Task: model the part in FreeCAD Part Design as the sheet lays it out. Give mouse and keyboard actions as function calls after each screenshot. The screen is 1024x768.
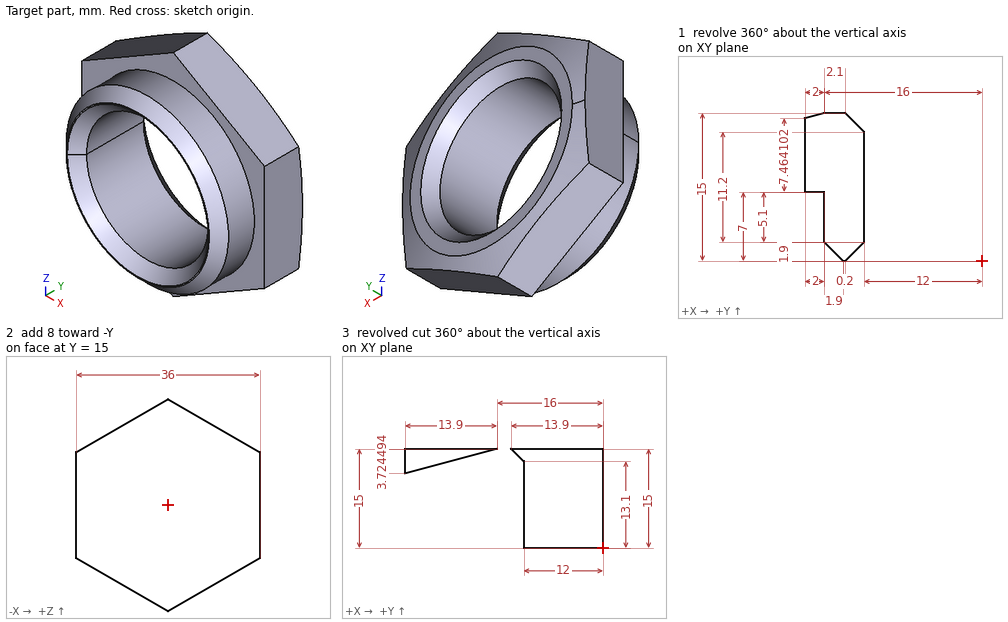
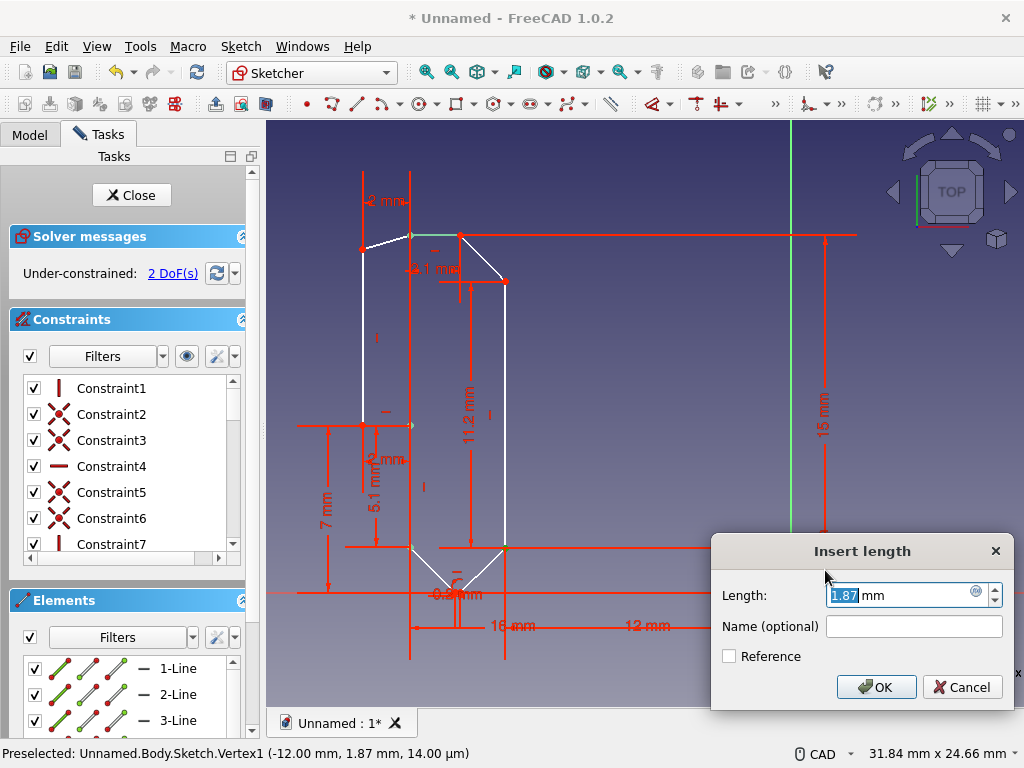
text(1.9)
key(Return)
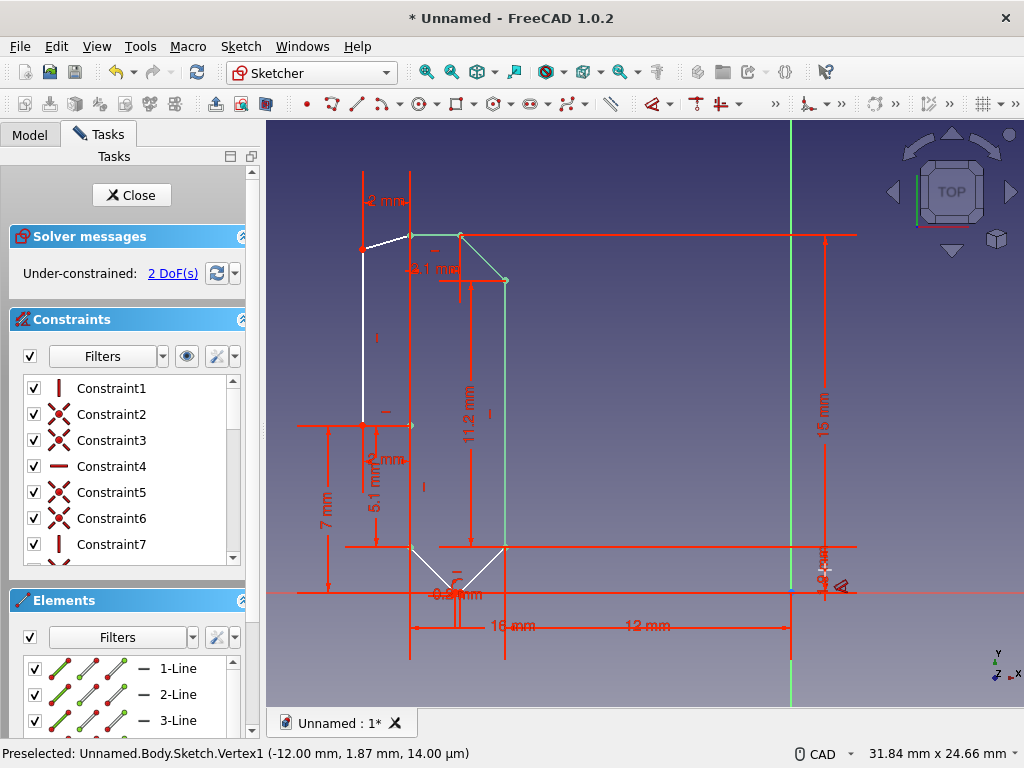
click(424, 561)
click(433, 627)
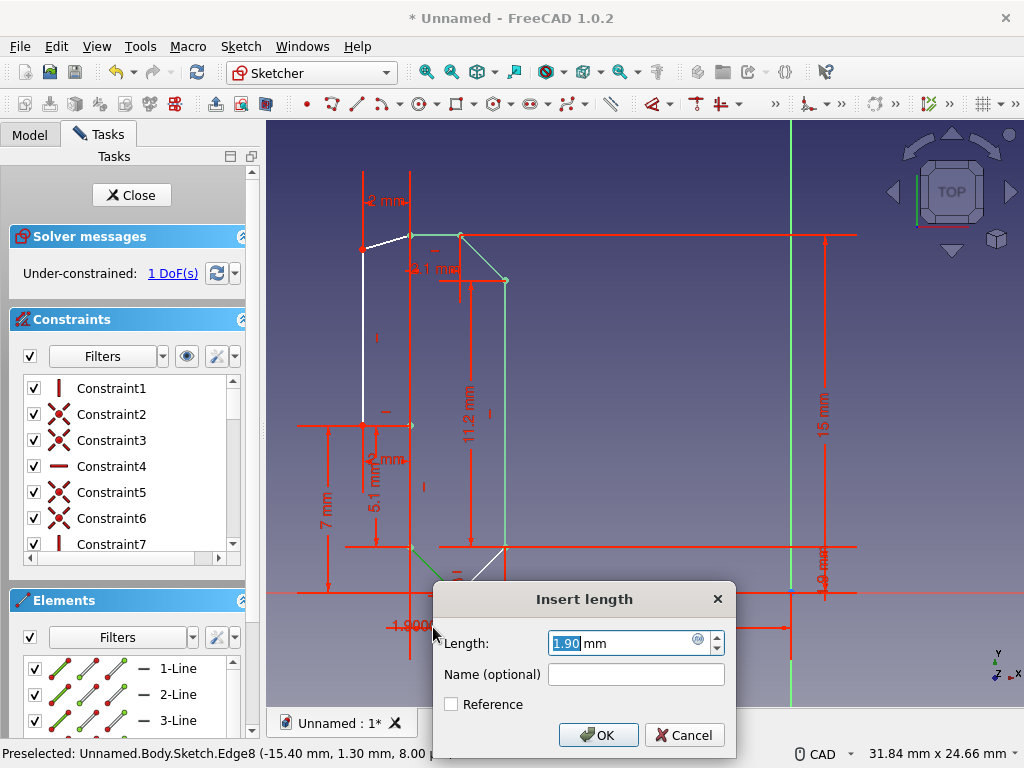
text(1.9)
key(Return)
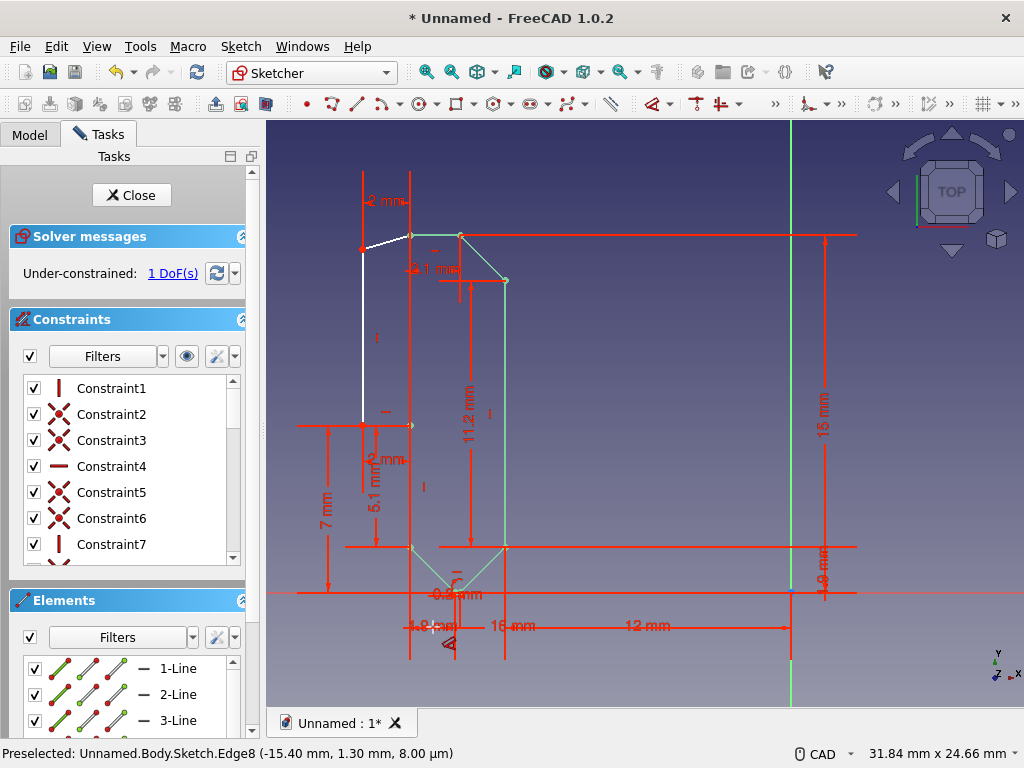
click(363, 302)
click(329, 338)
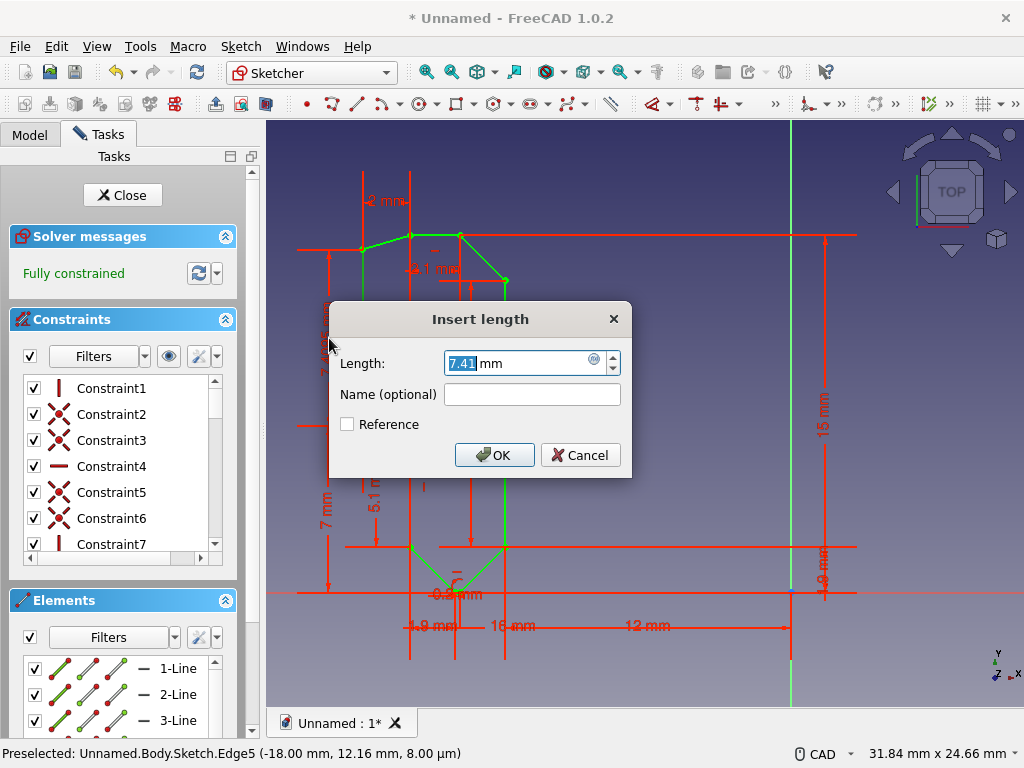
text(7.464102)
key(Return)
key(Escape)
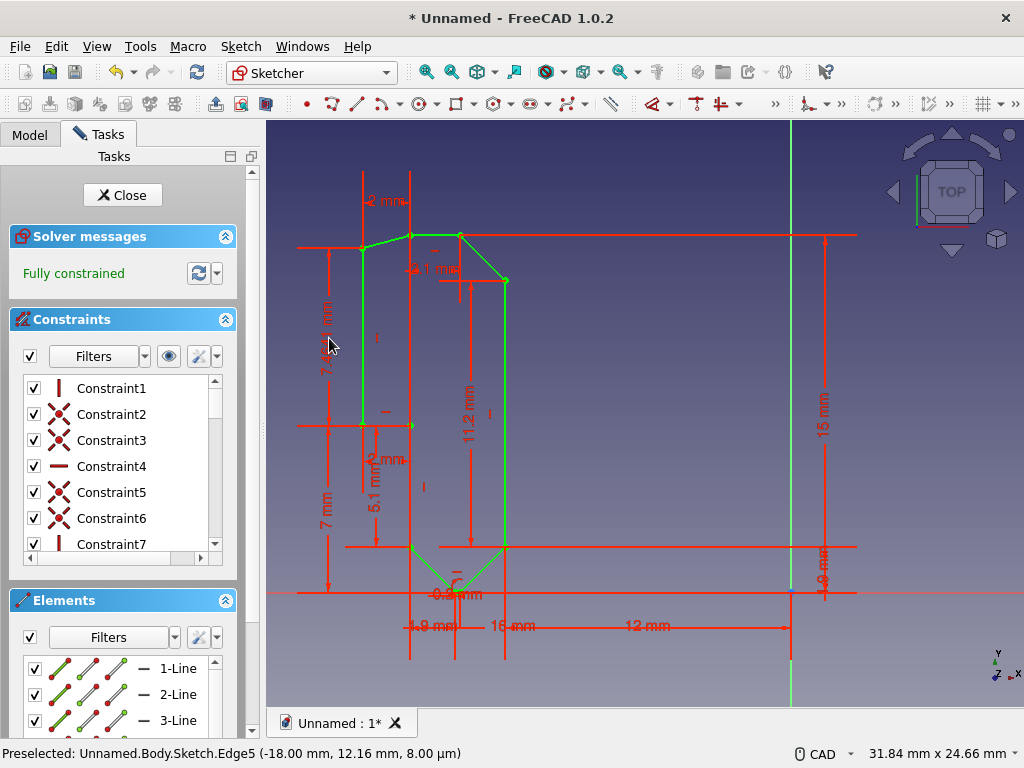
click(123, 195)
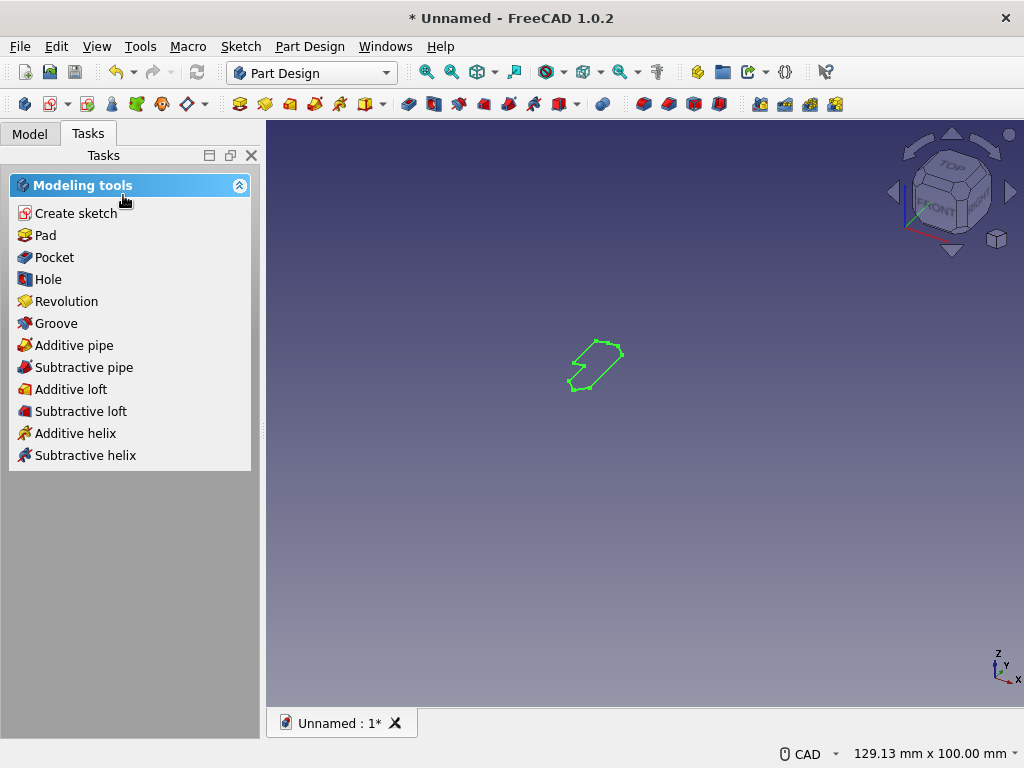
click(265, 104)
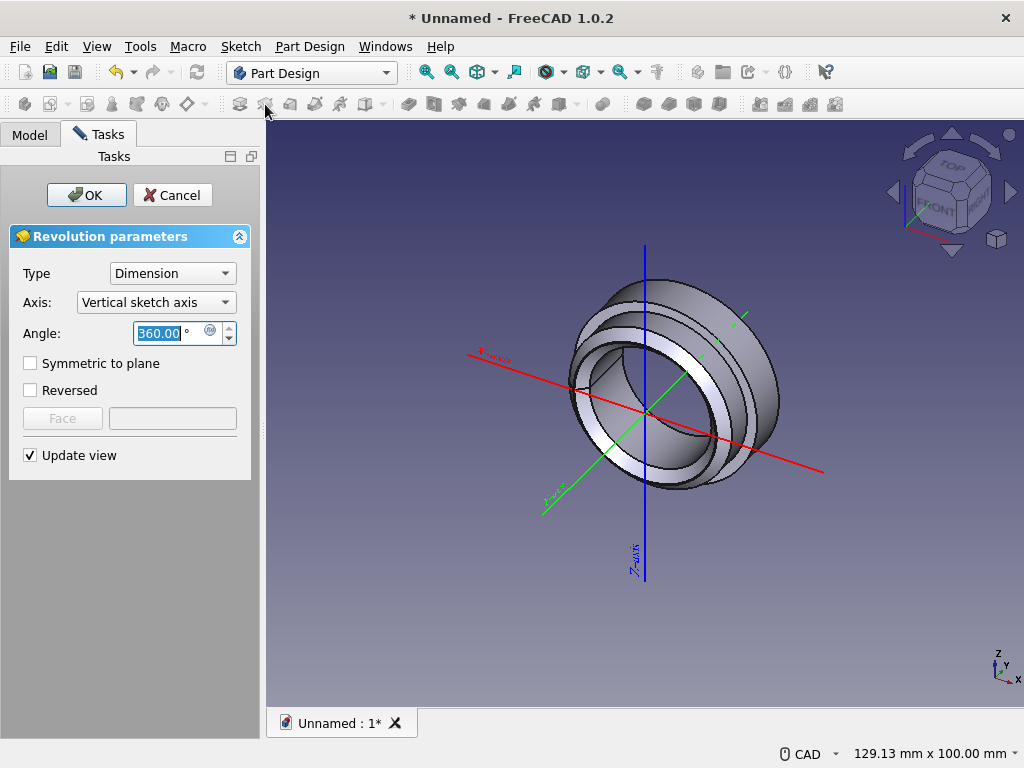
click(87, 195)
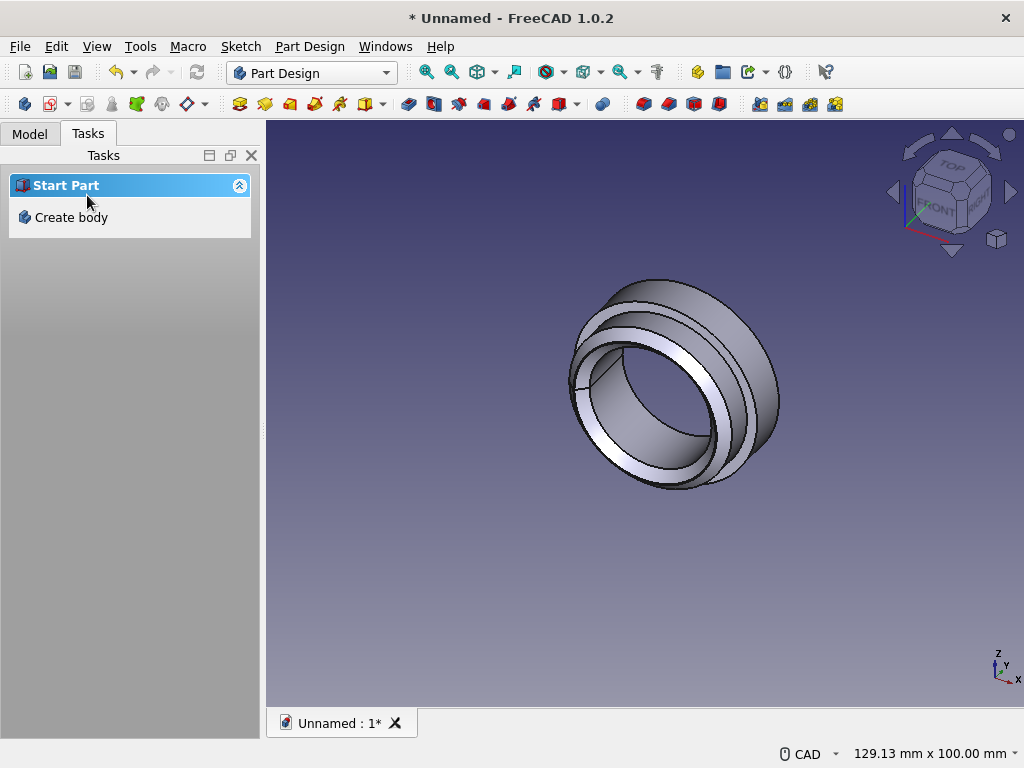
key(4)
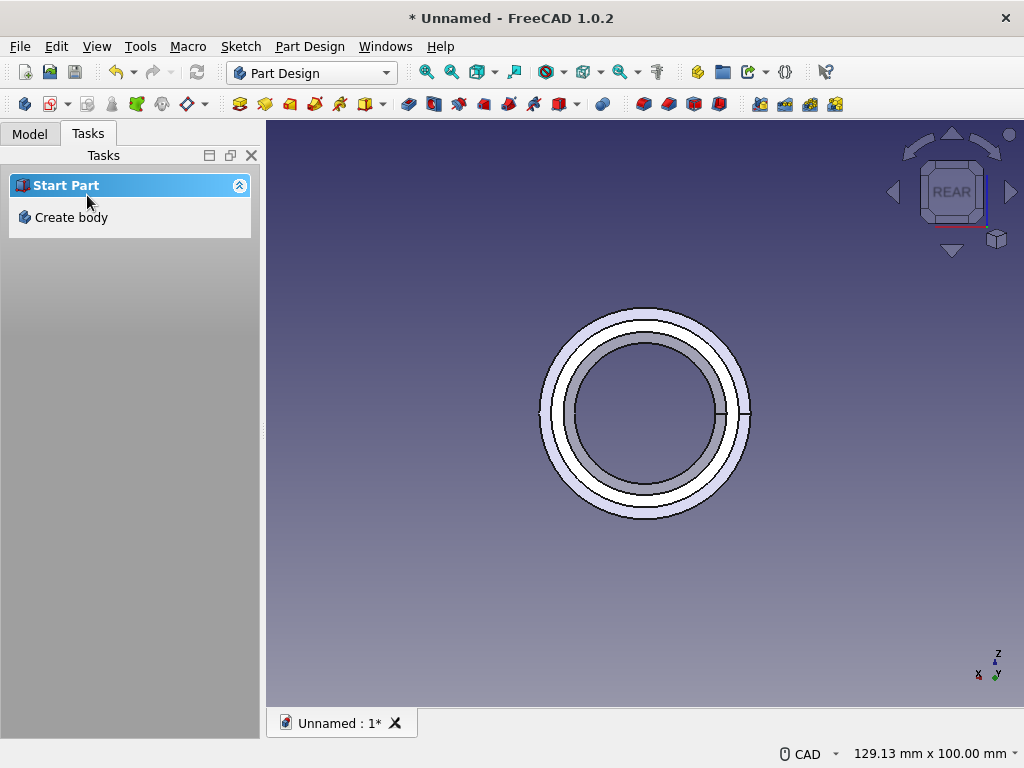
key(v)
key(f)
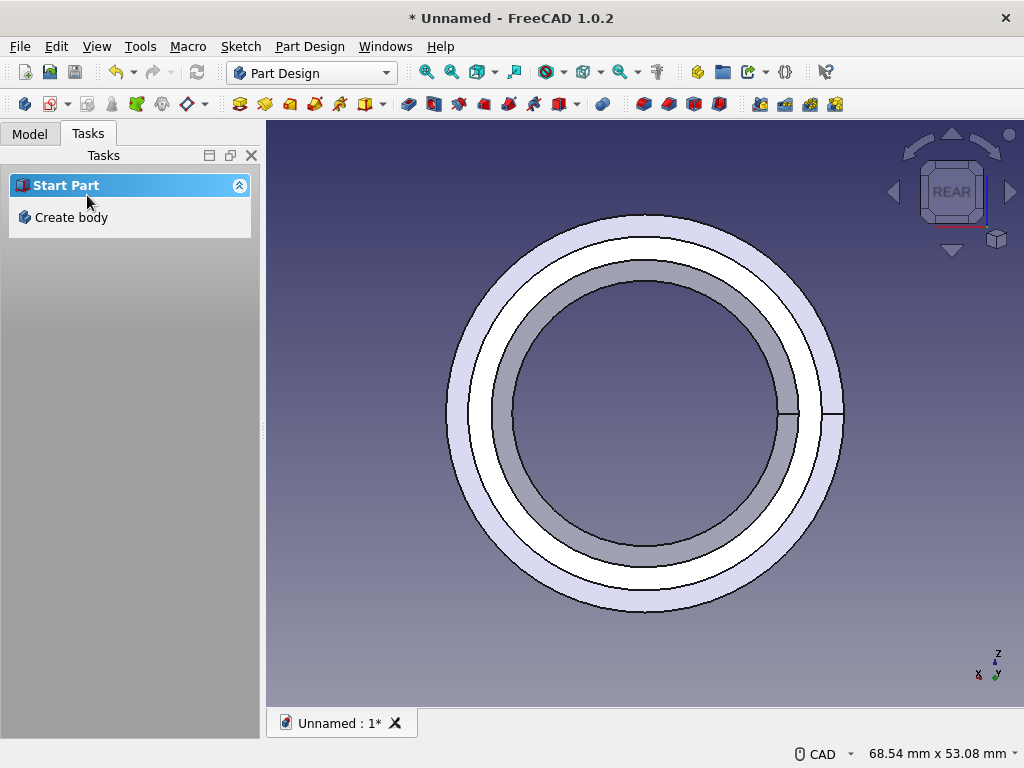
scroll(493, 362, up, 4)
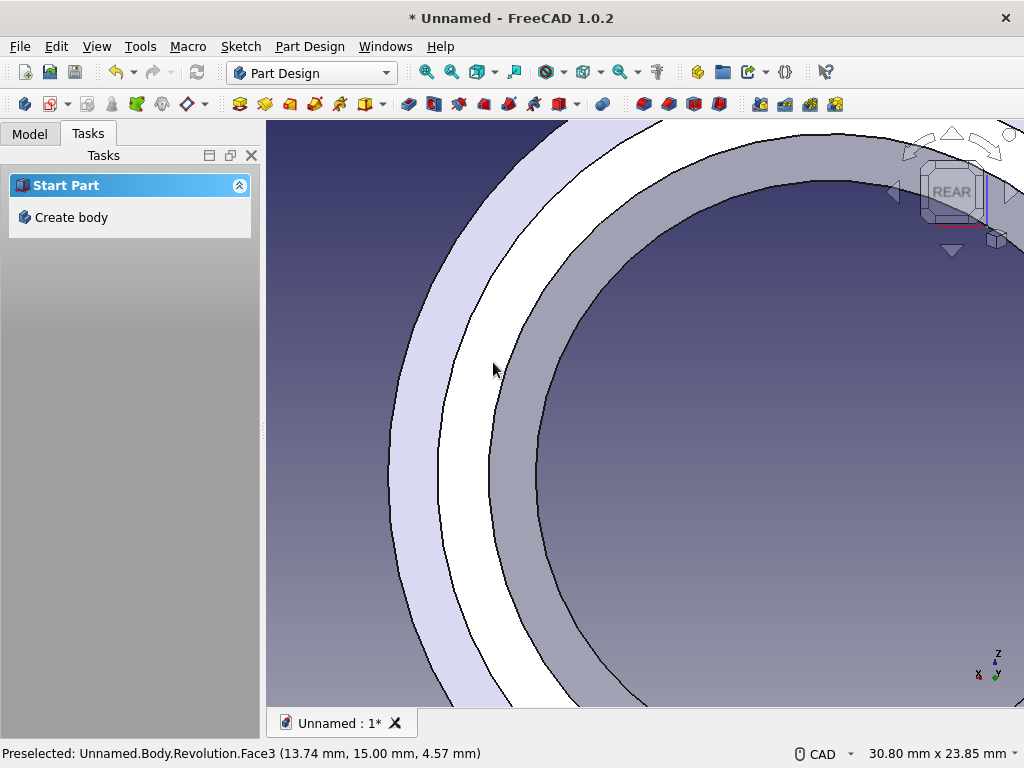
click(493, 363)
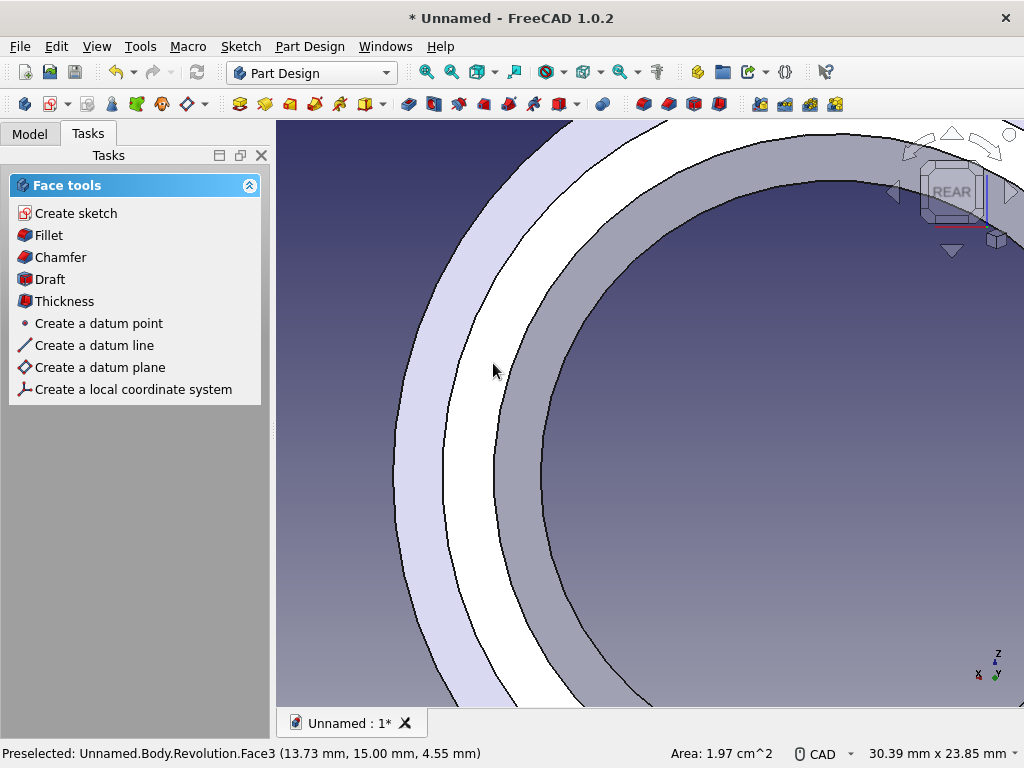
click(50, 104)